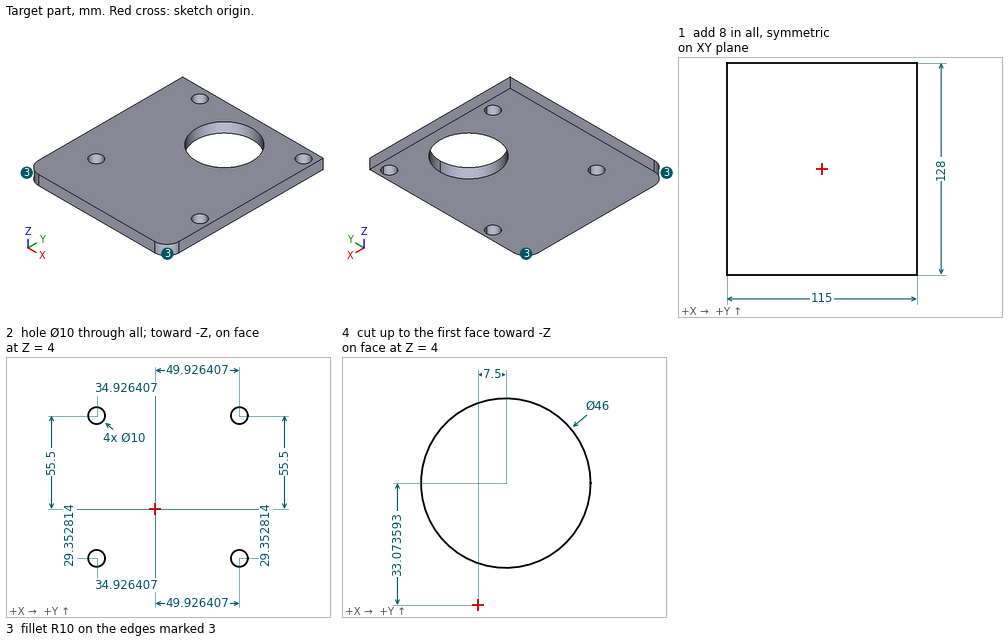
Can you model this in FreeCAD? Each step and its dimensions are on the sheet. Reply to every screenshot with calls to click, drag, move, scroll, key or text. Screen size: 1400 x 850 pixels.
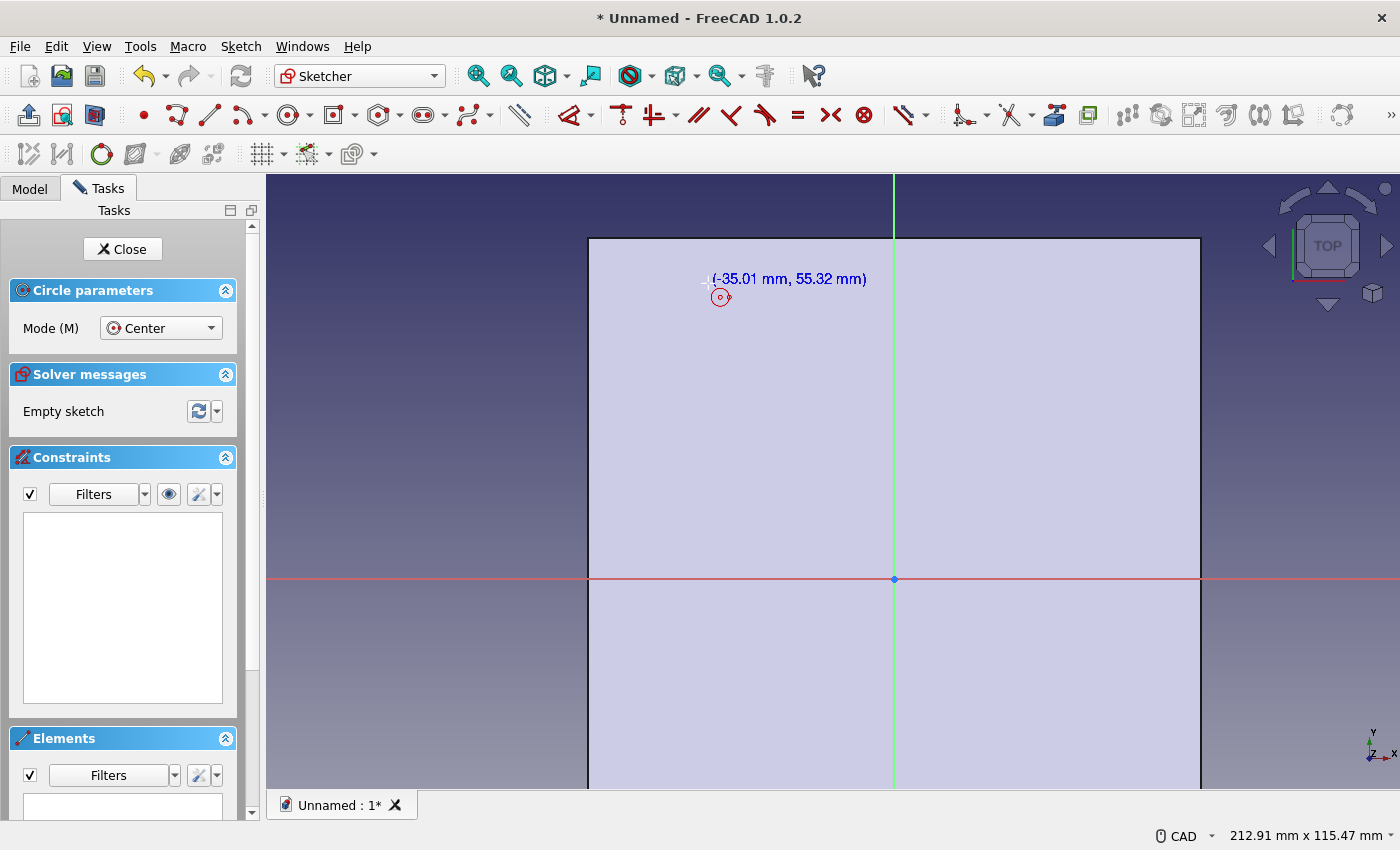
click(708, 283)
move(727, 265)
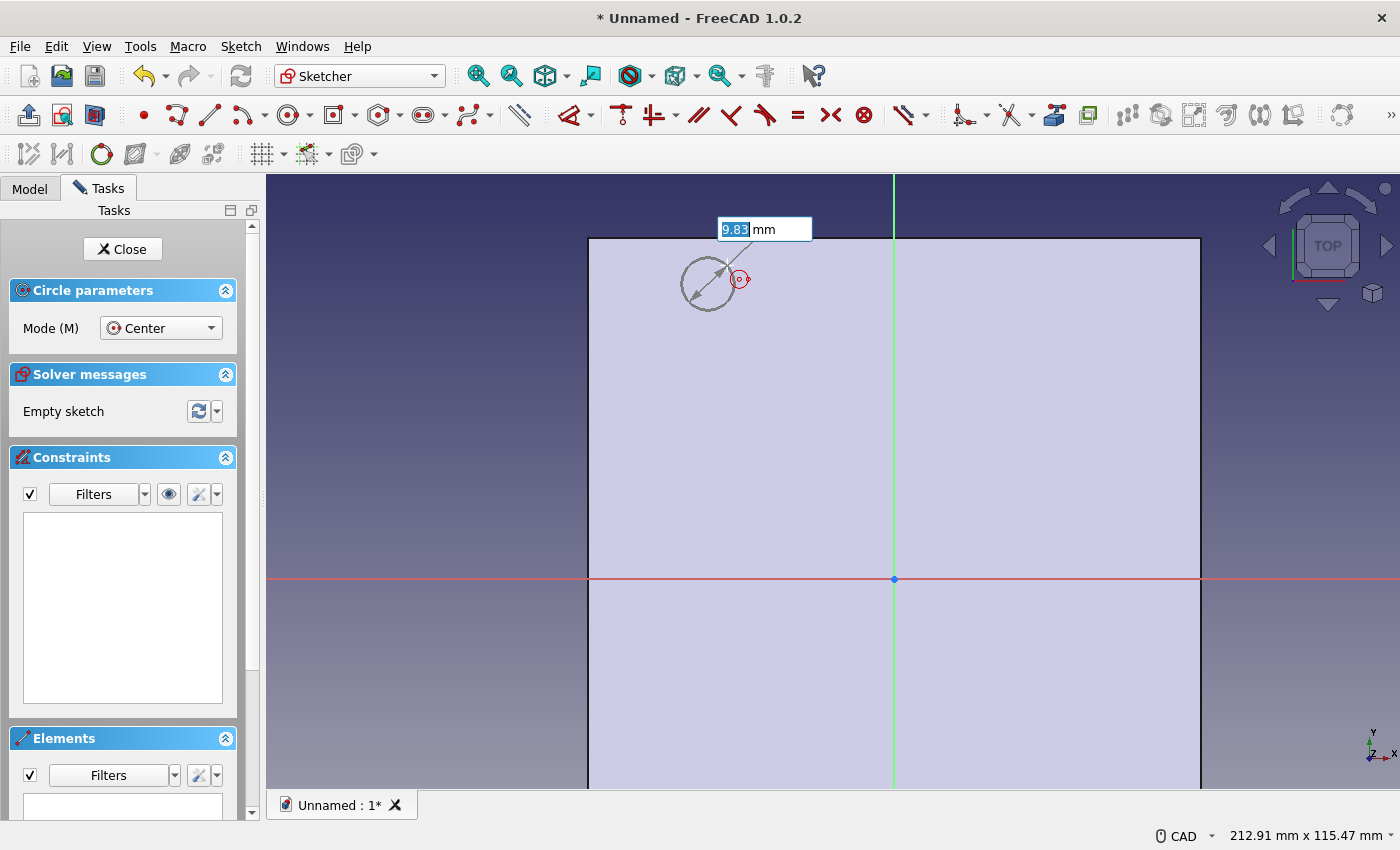
text(10)
key(Return)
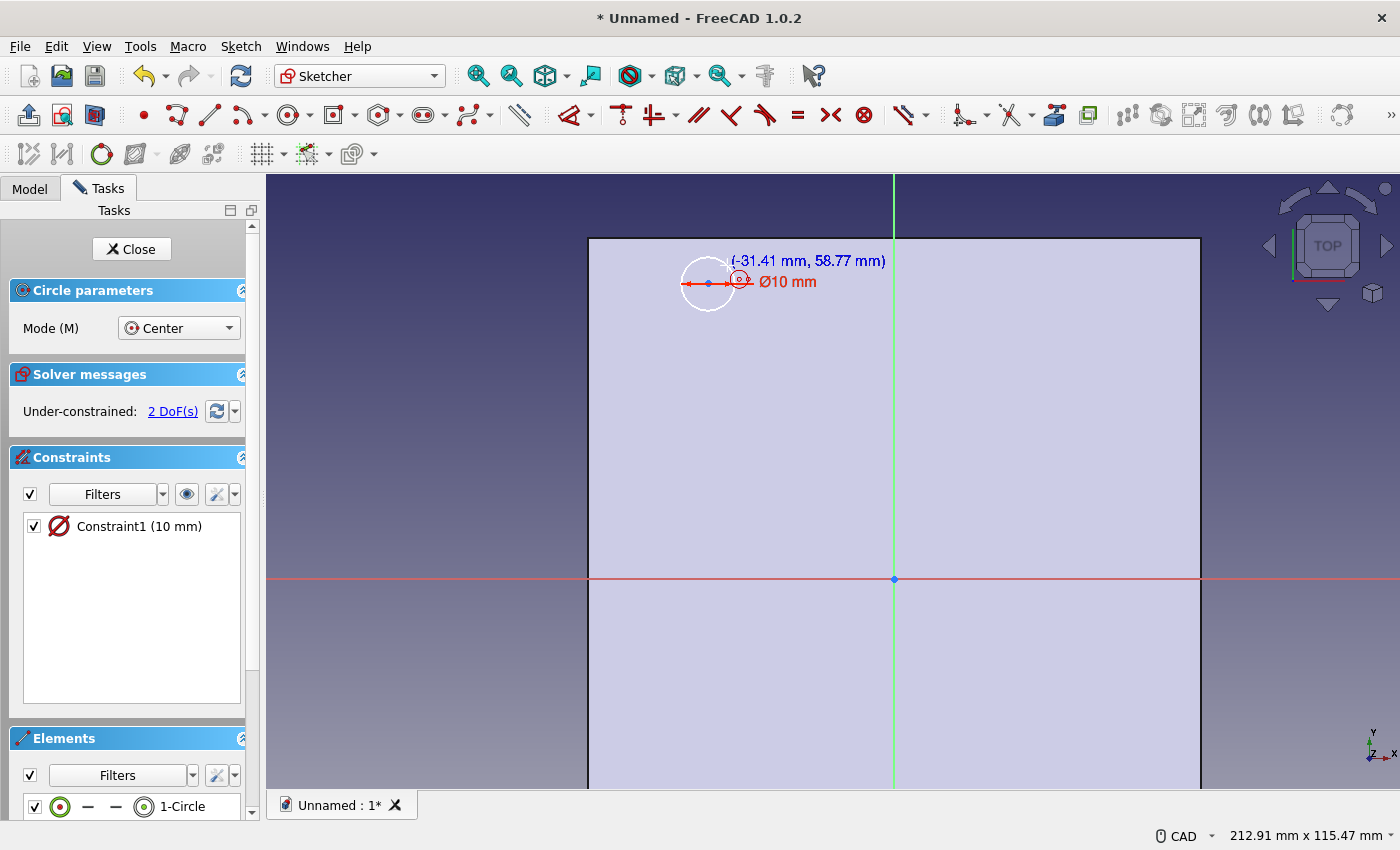
click(1160, 283)
move(1179, 265)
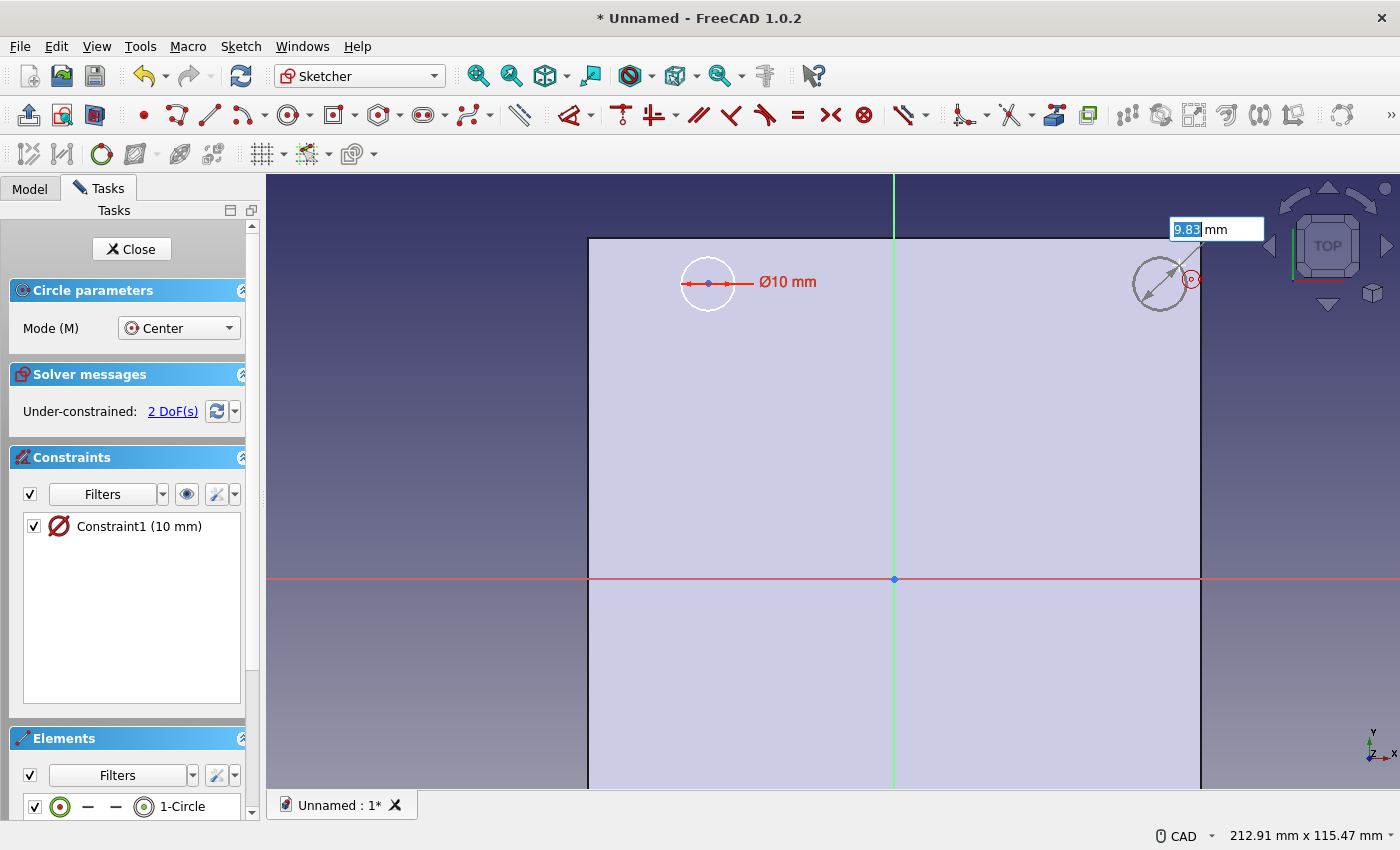
text(10)
key(Return)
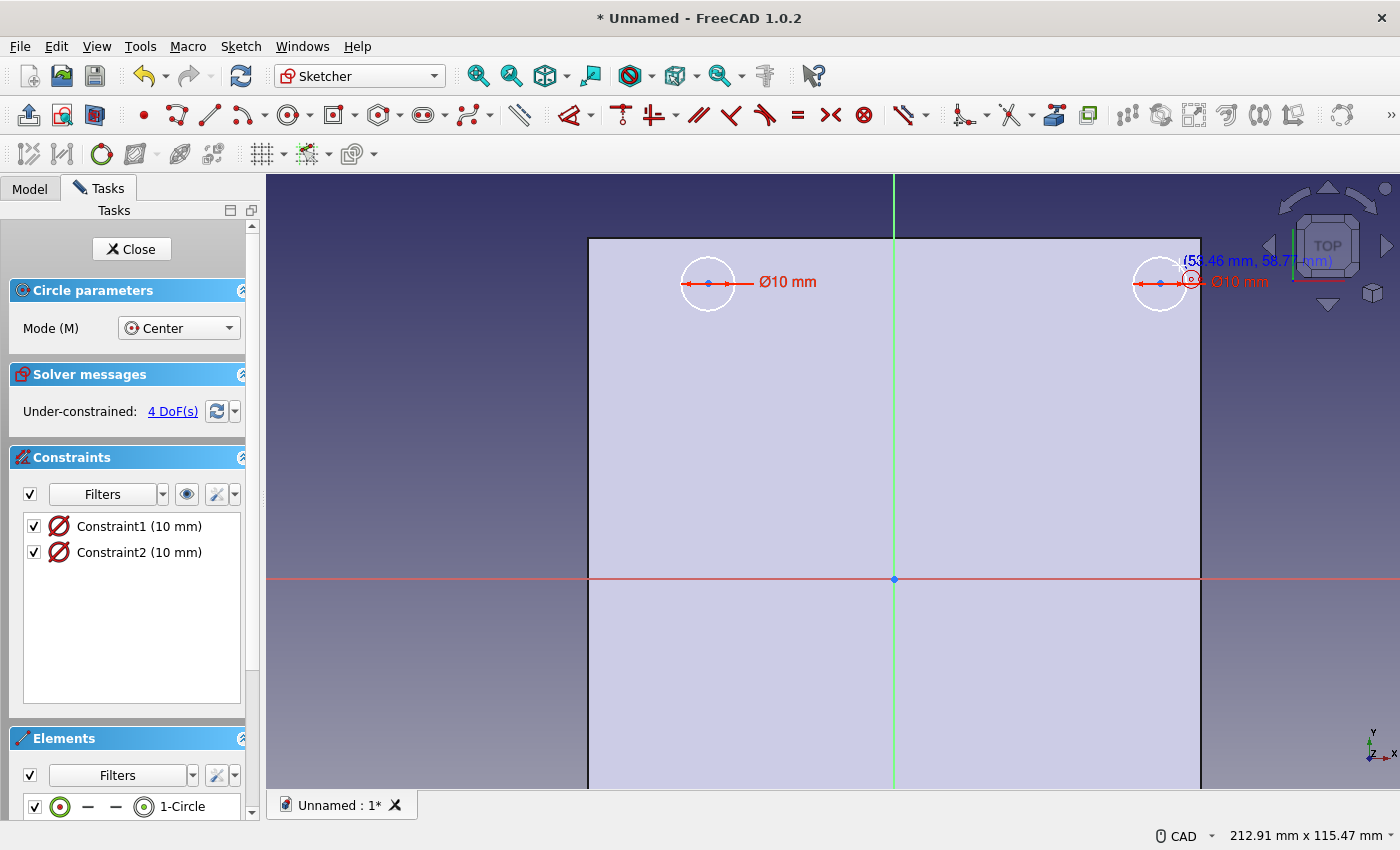
click(1160, 735)
move(1179, 717)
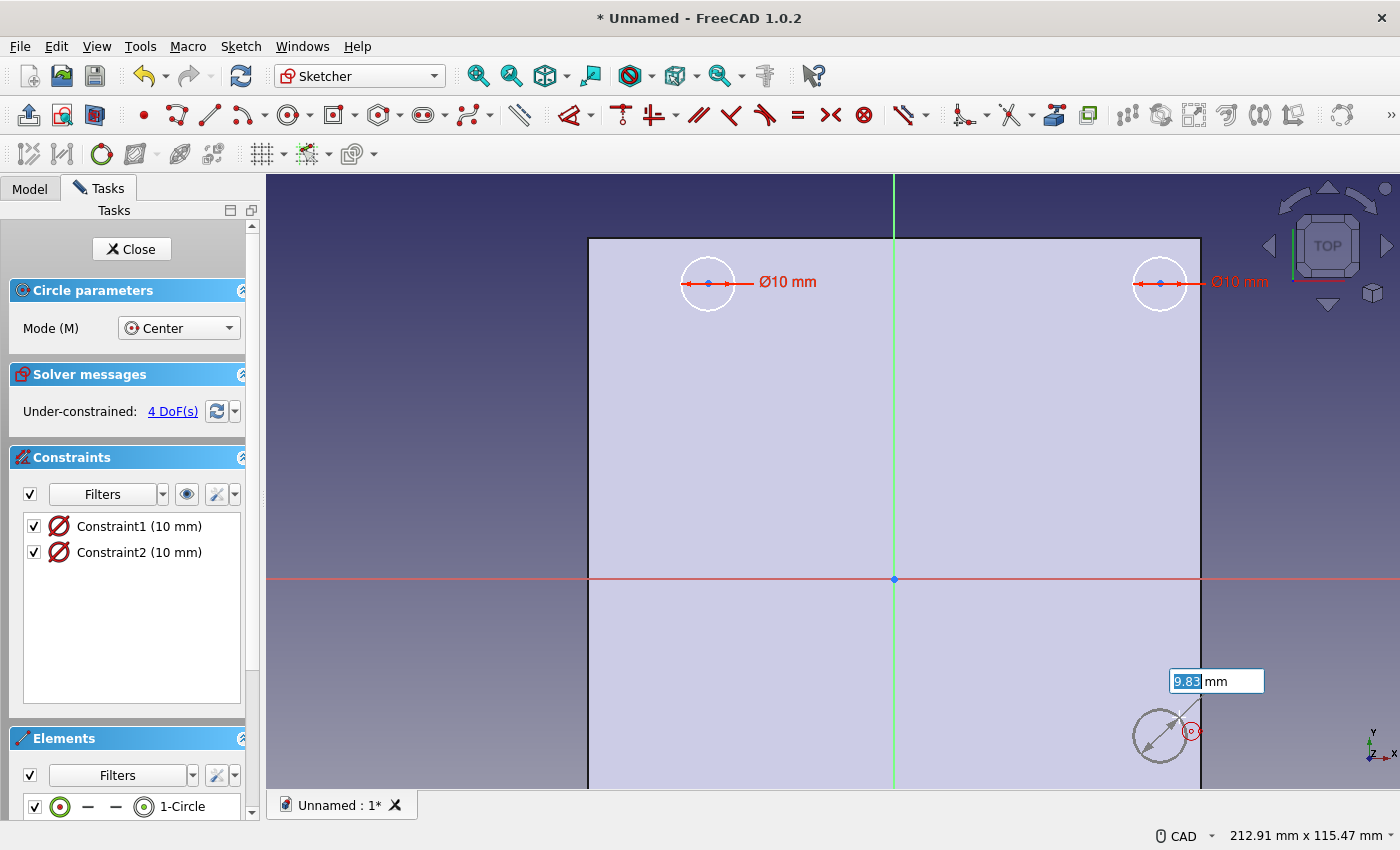
text(10)
key(Return)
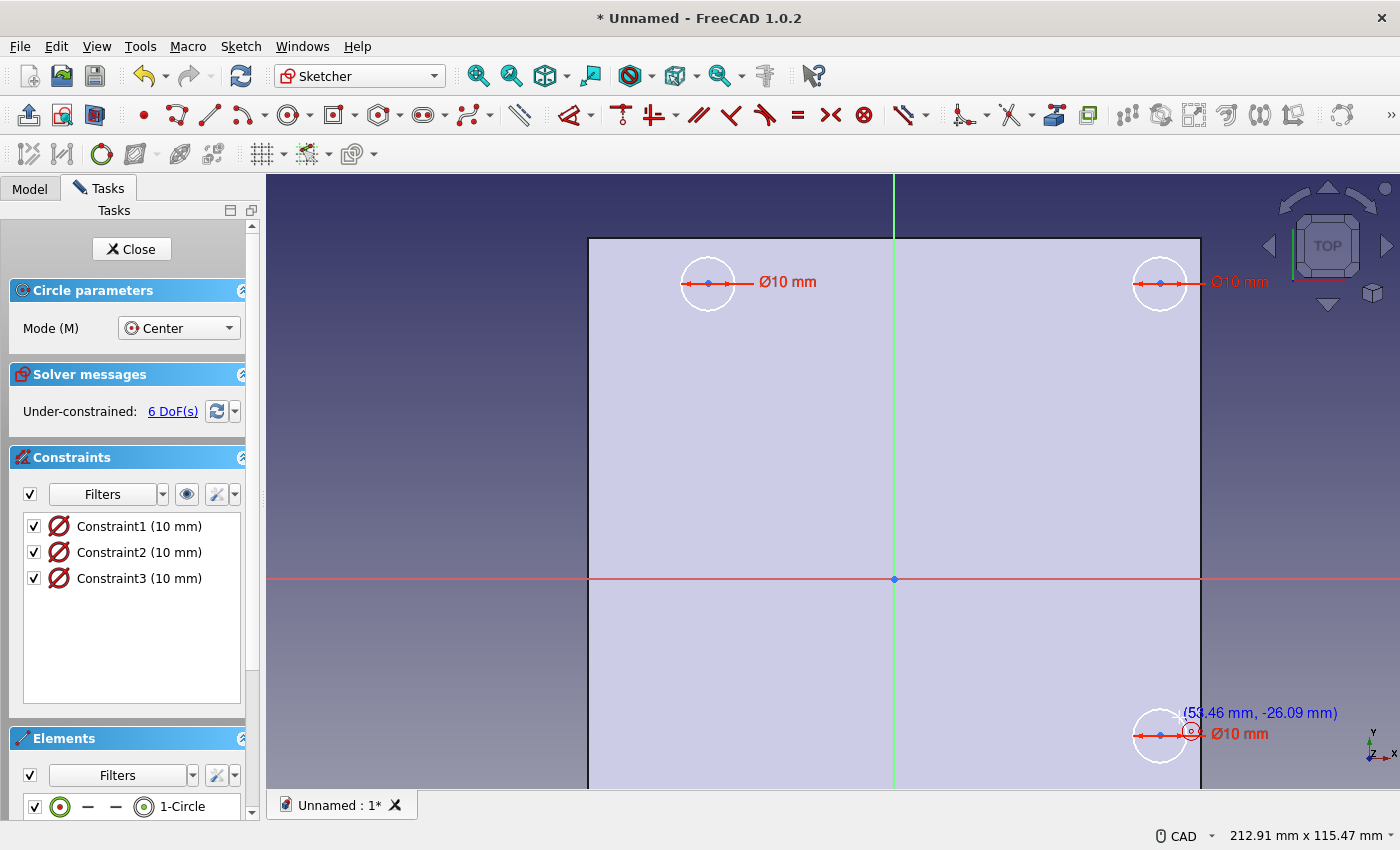
click(708, 735)
move(727, 717)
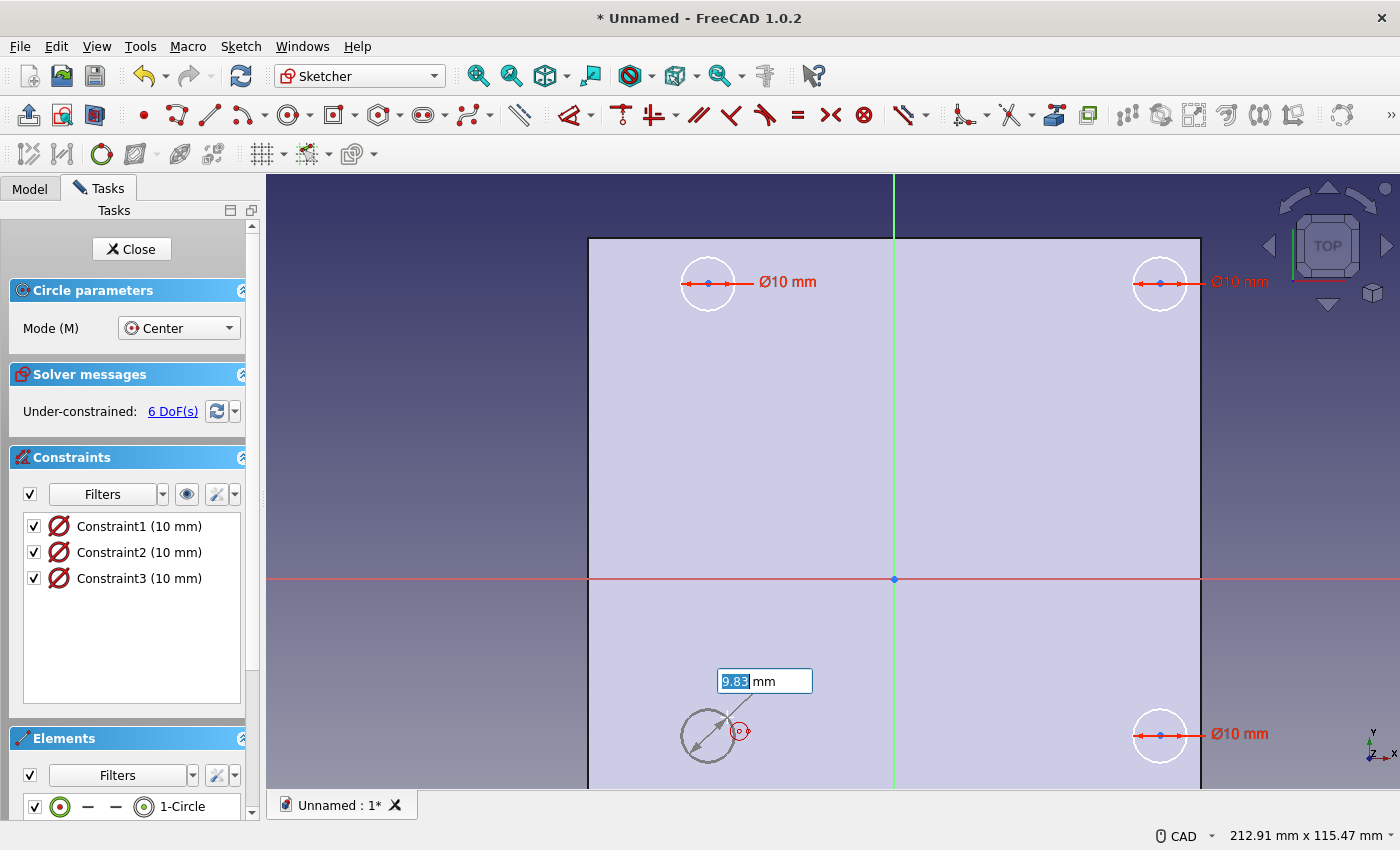
text(10)
key(Return)
key(Escape)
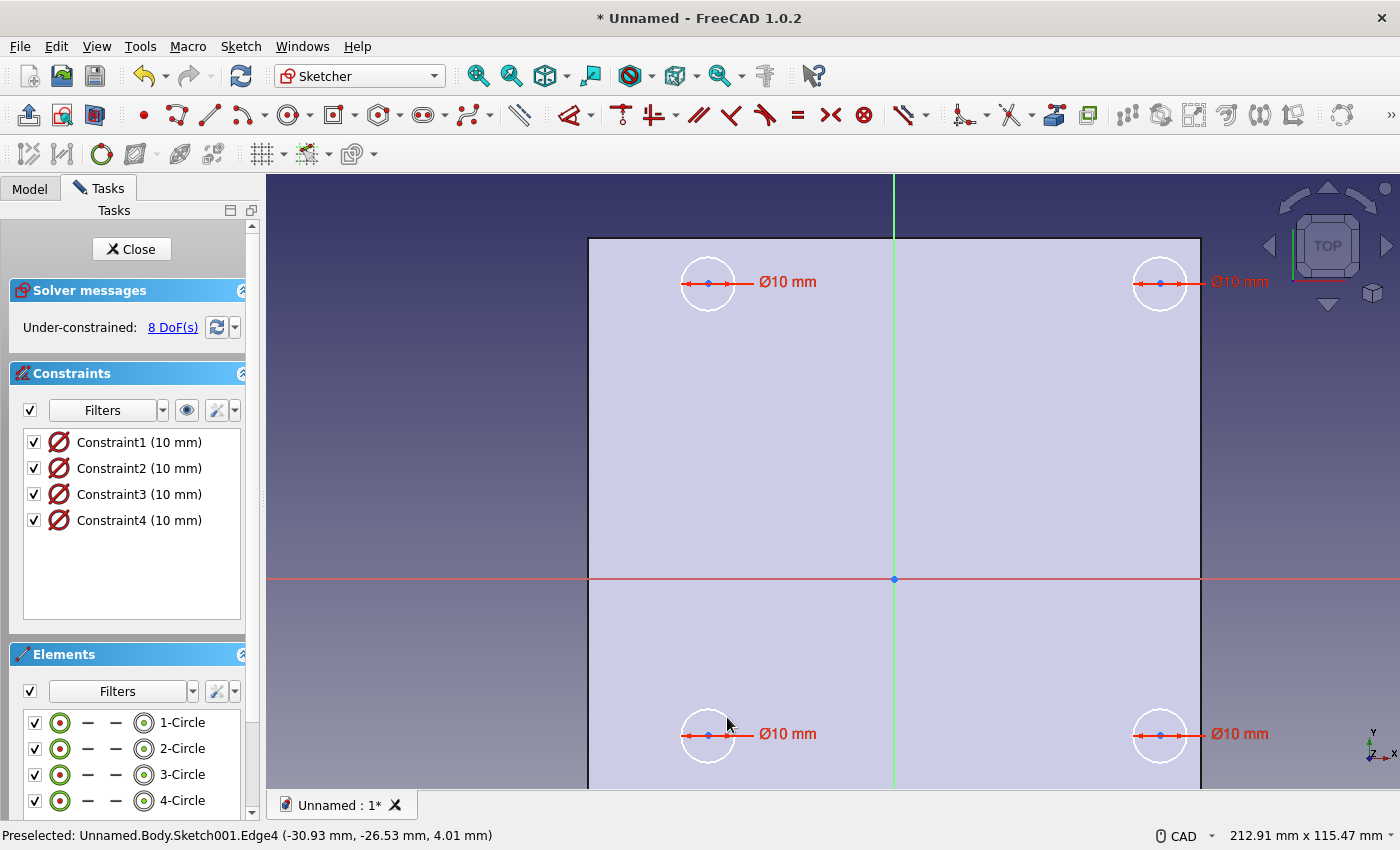
click(568, 116)